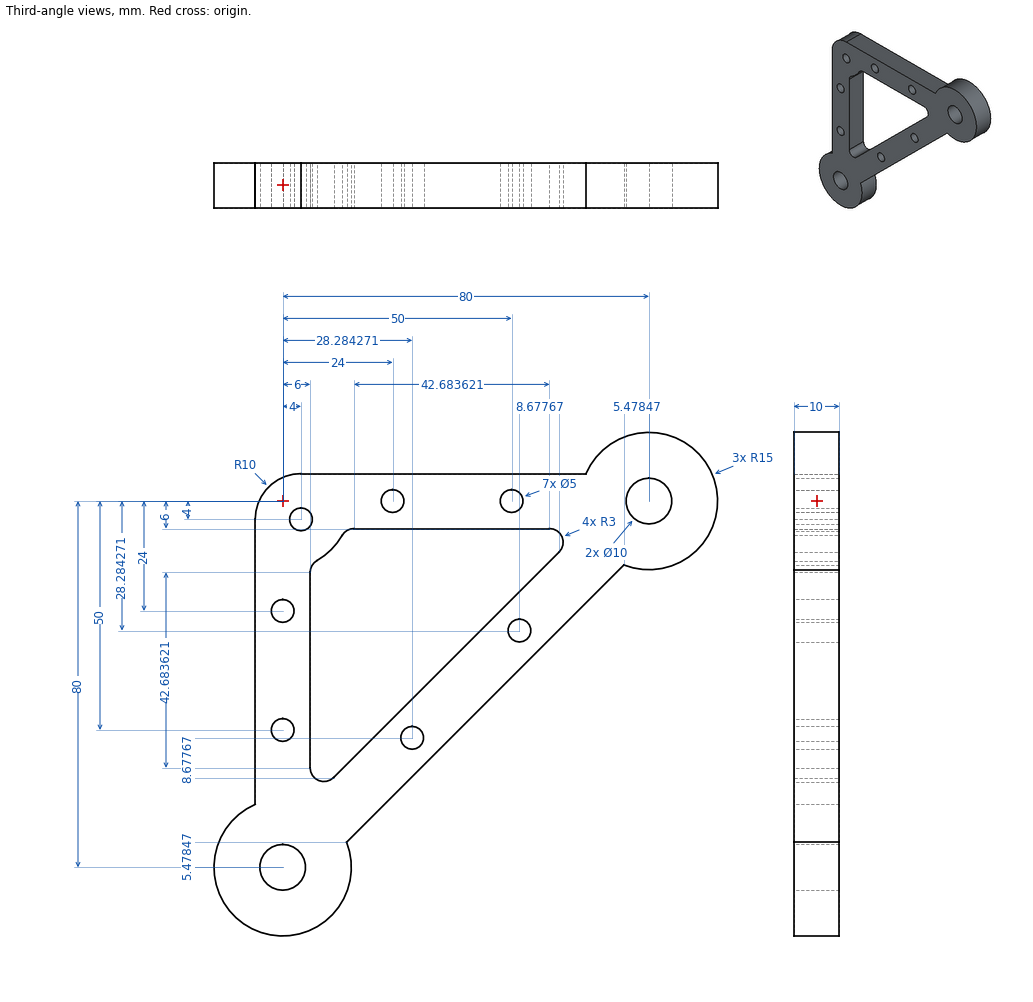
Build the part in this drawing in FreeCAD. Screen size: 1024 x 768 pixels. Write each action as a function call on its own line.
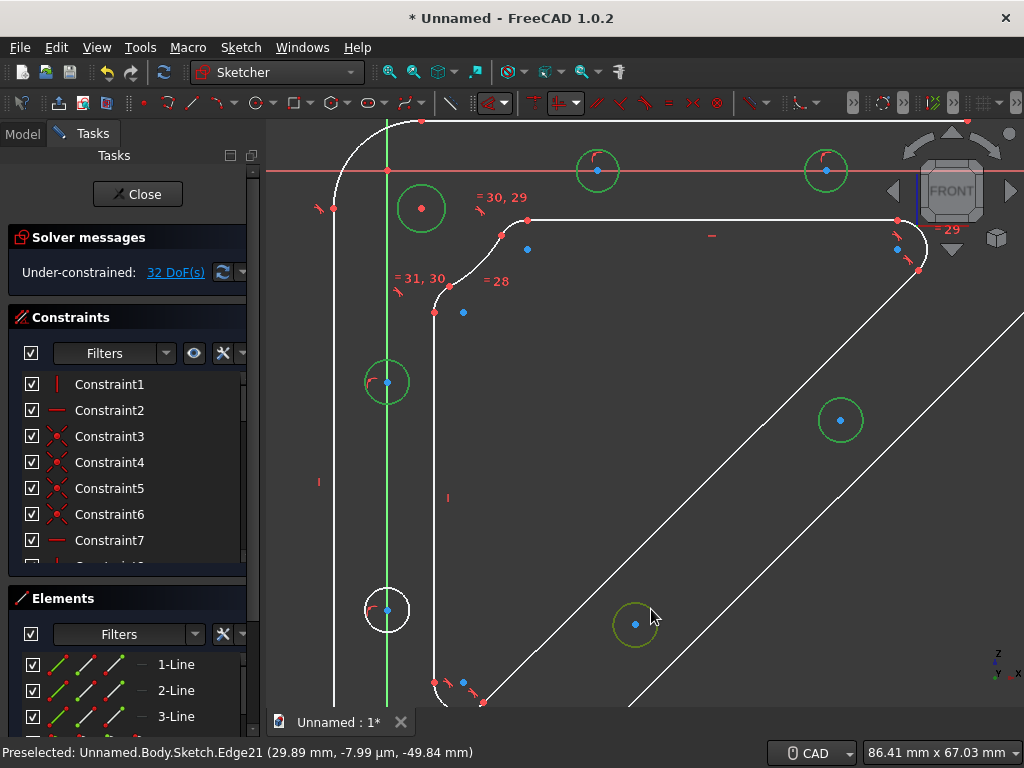
click(403, 594)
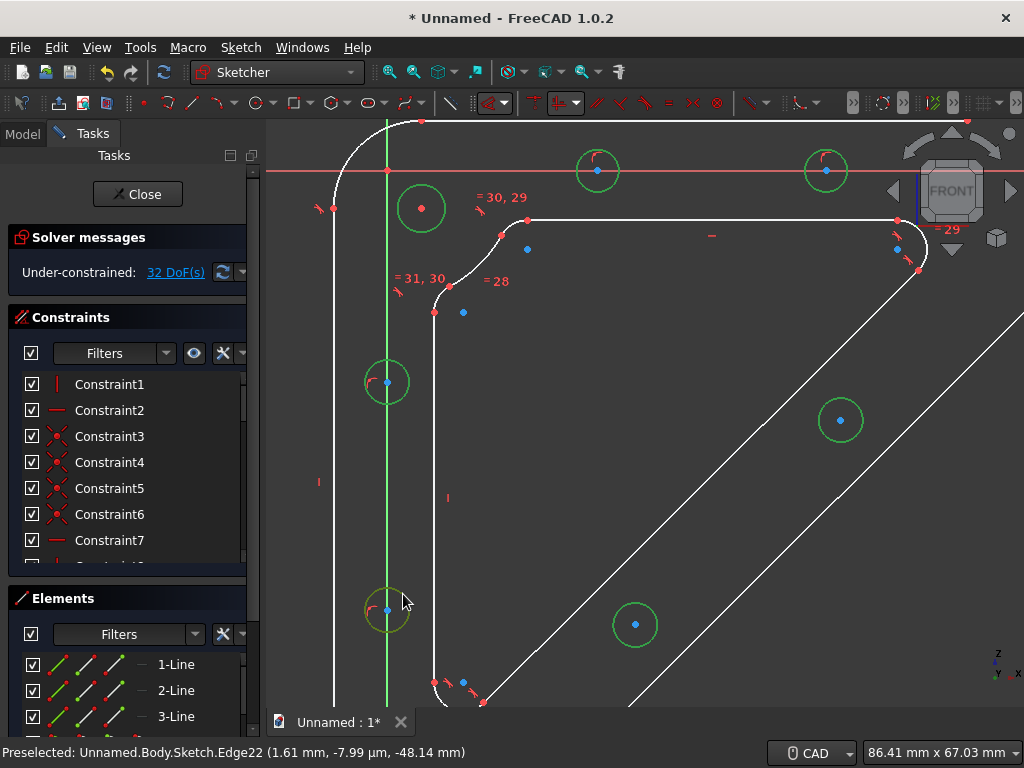
click(670, 104)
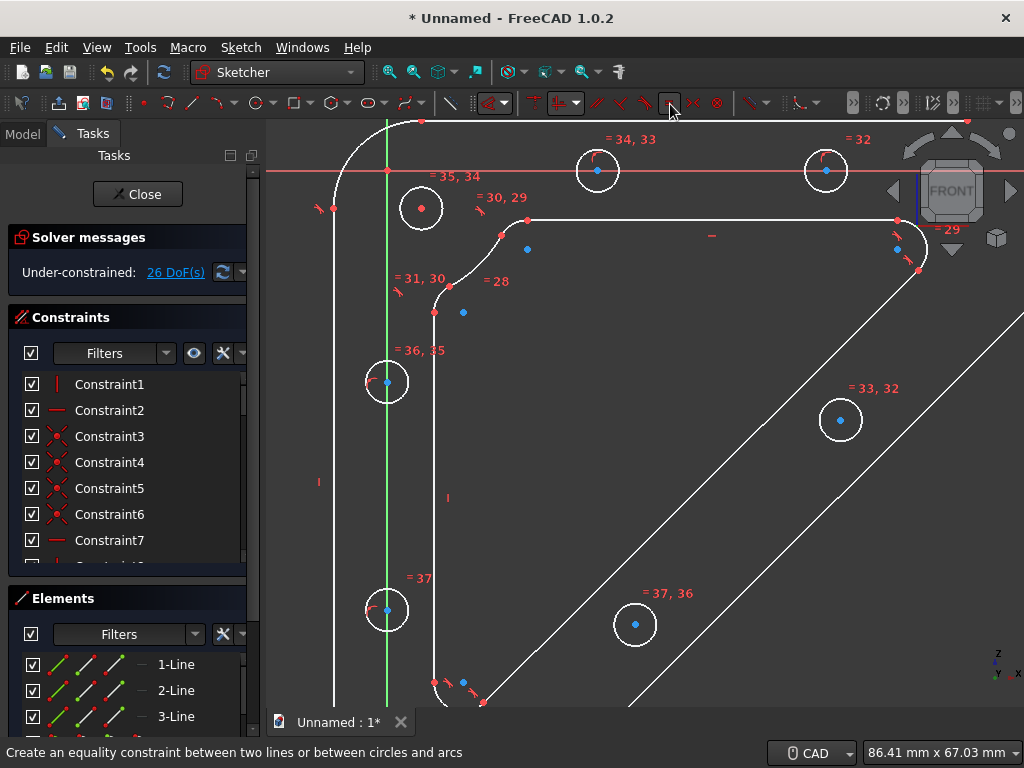
scroll(417, 296, down, 4)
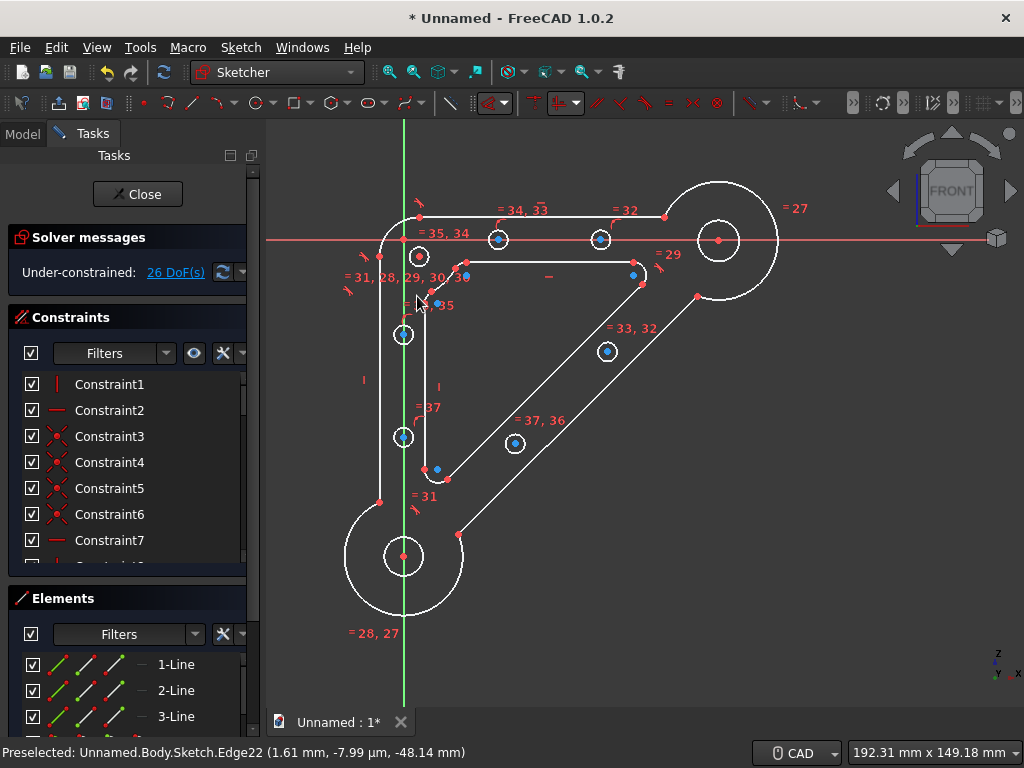
click(733, 226)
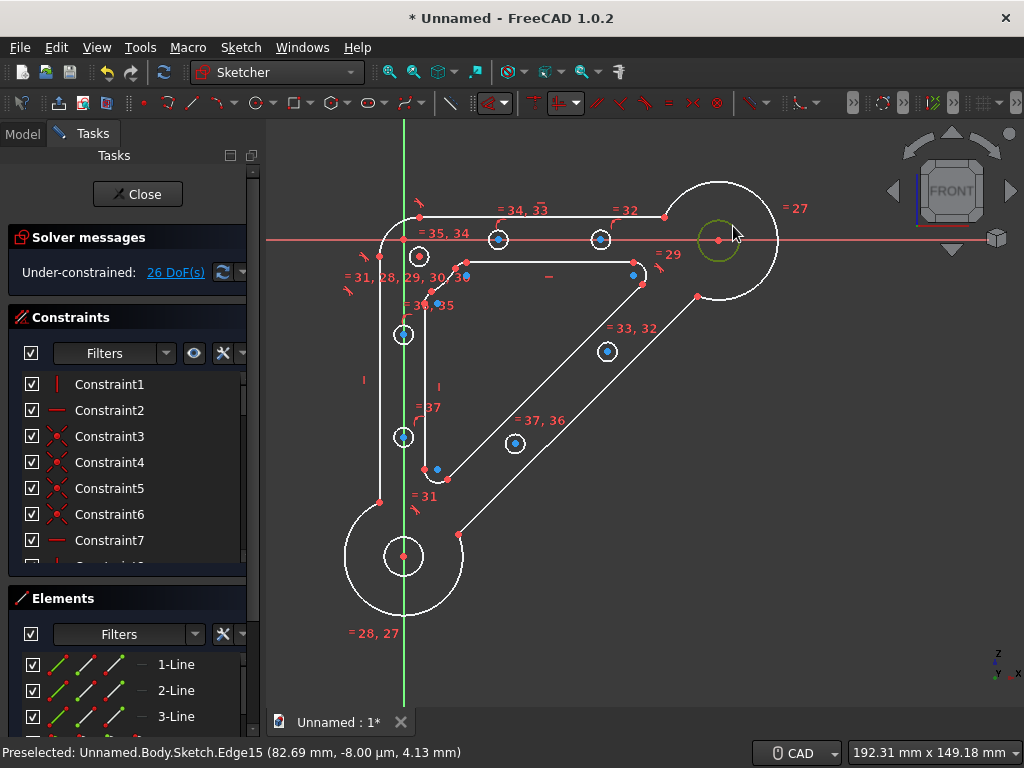
click(417, 543)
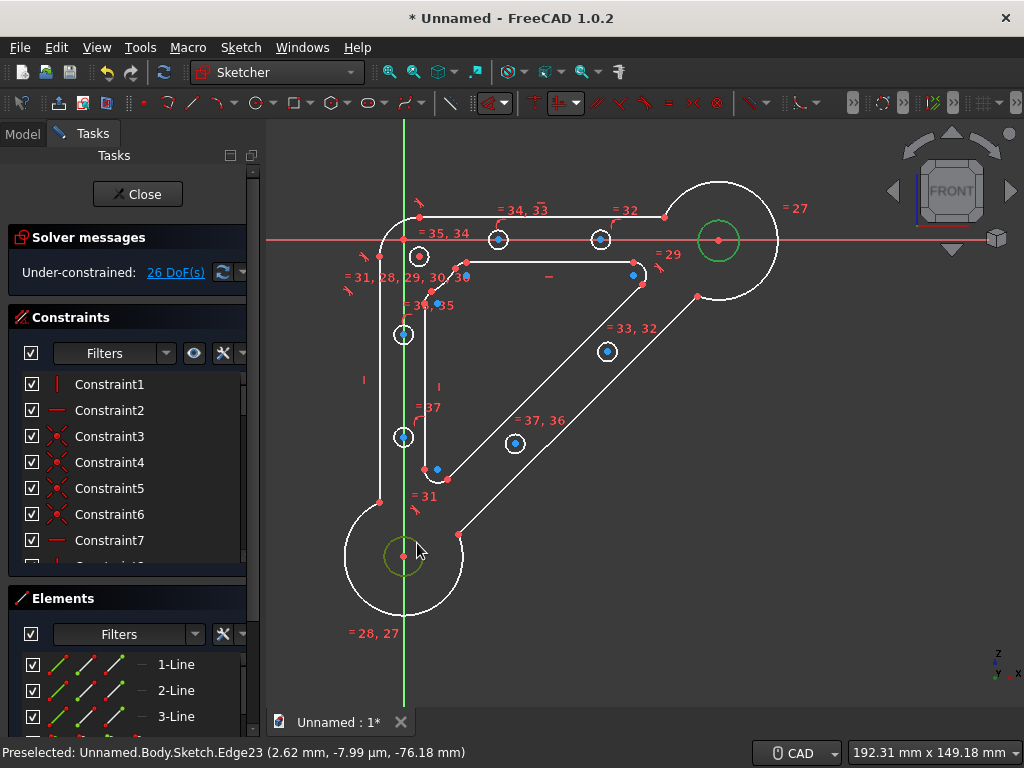
click(670, 104)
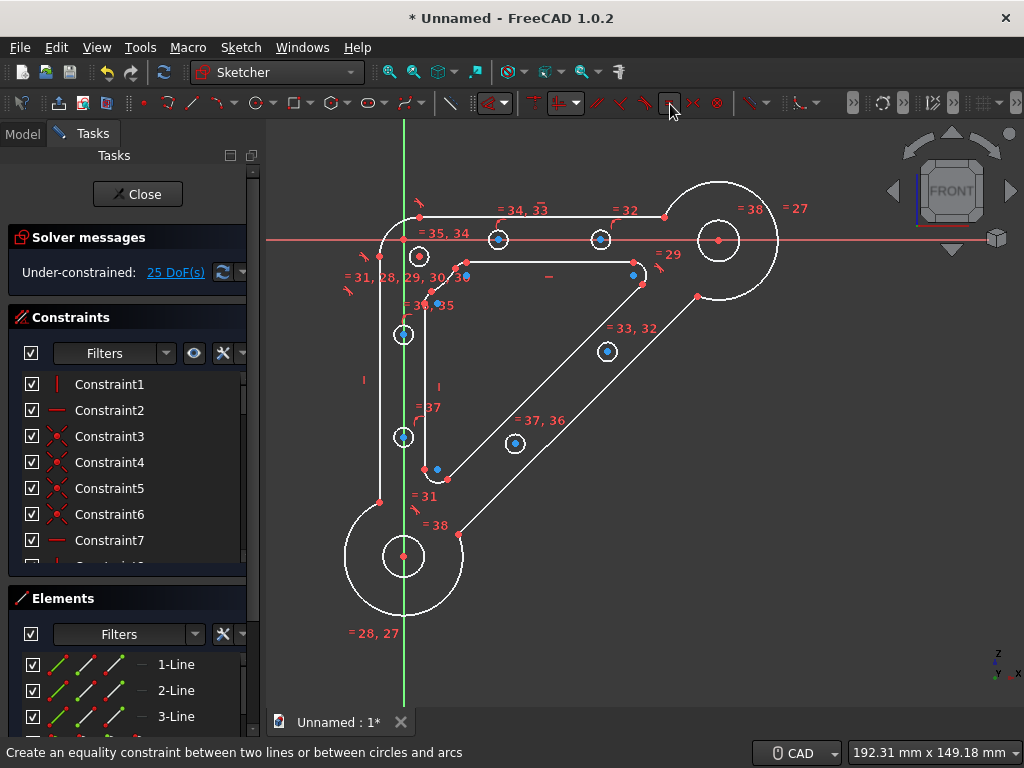
click(719, 241)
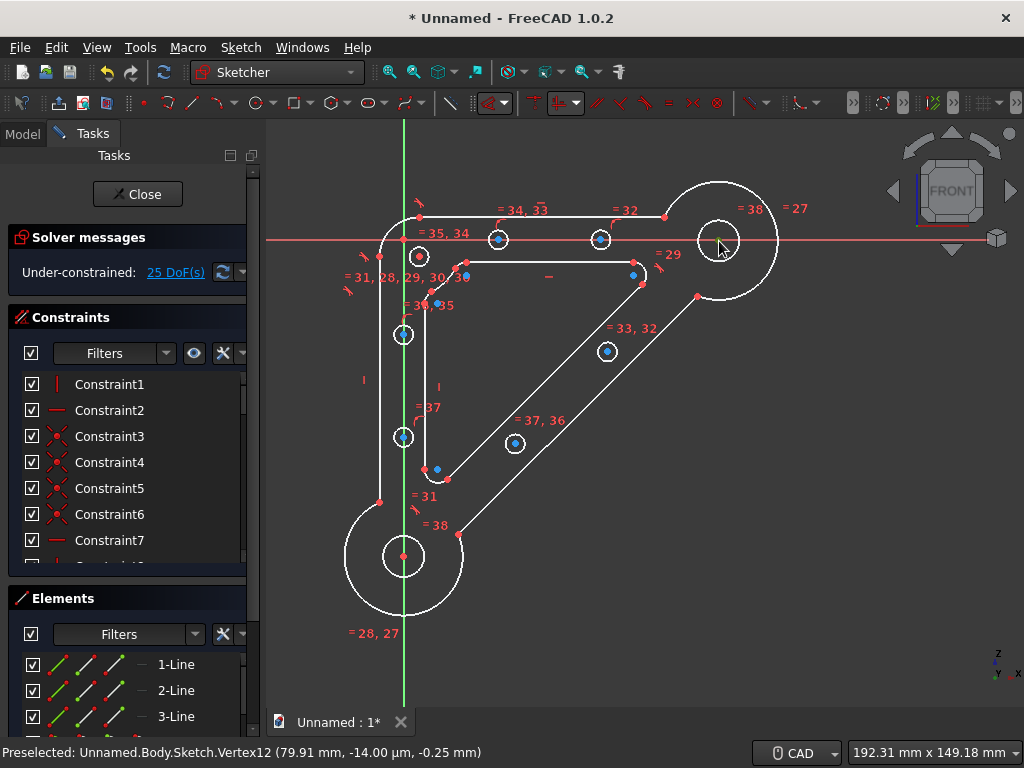
click(334, 240)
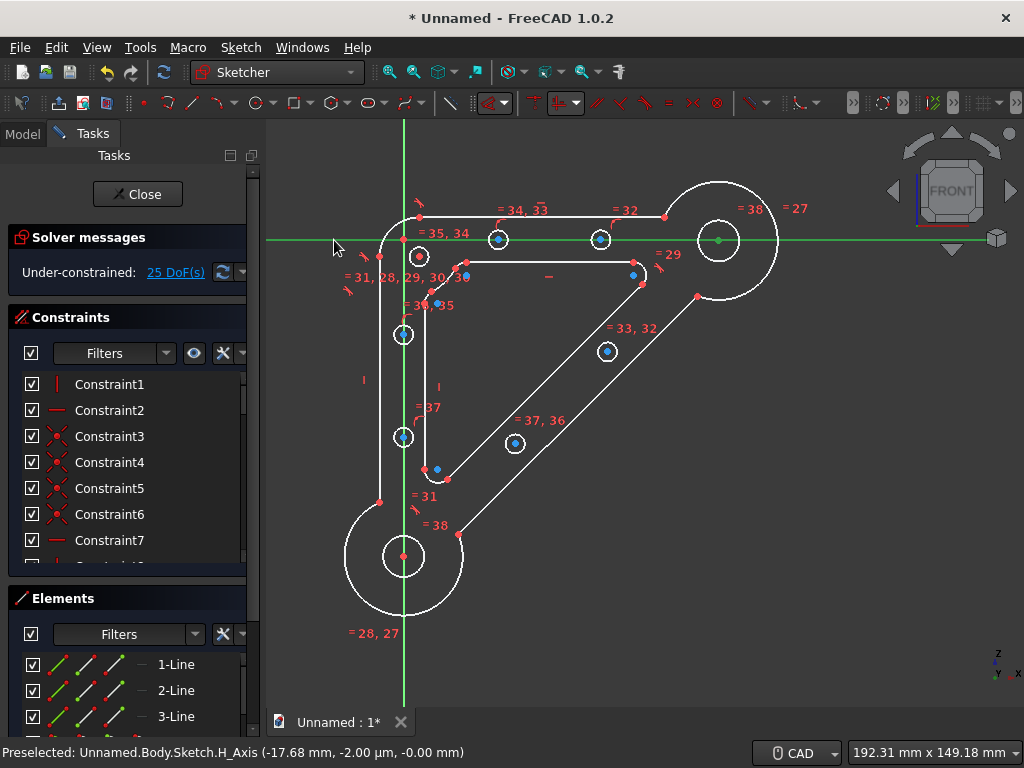
key(c)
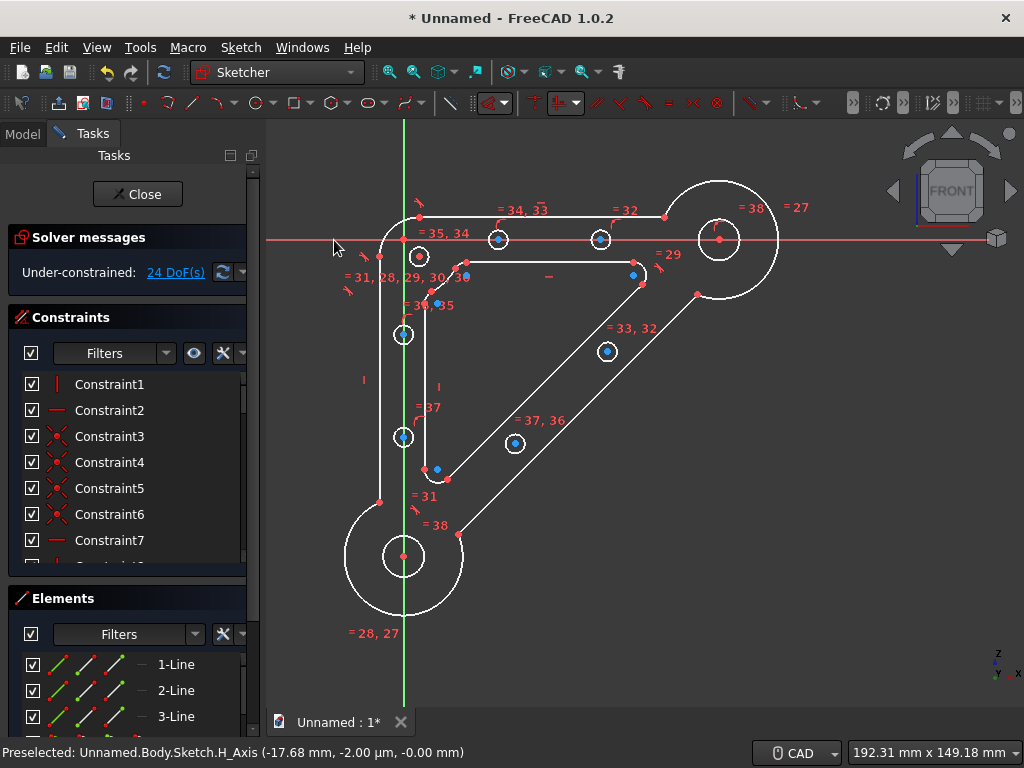
click(404, 557)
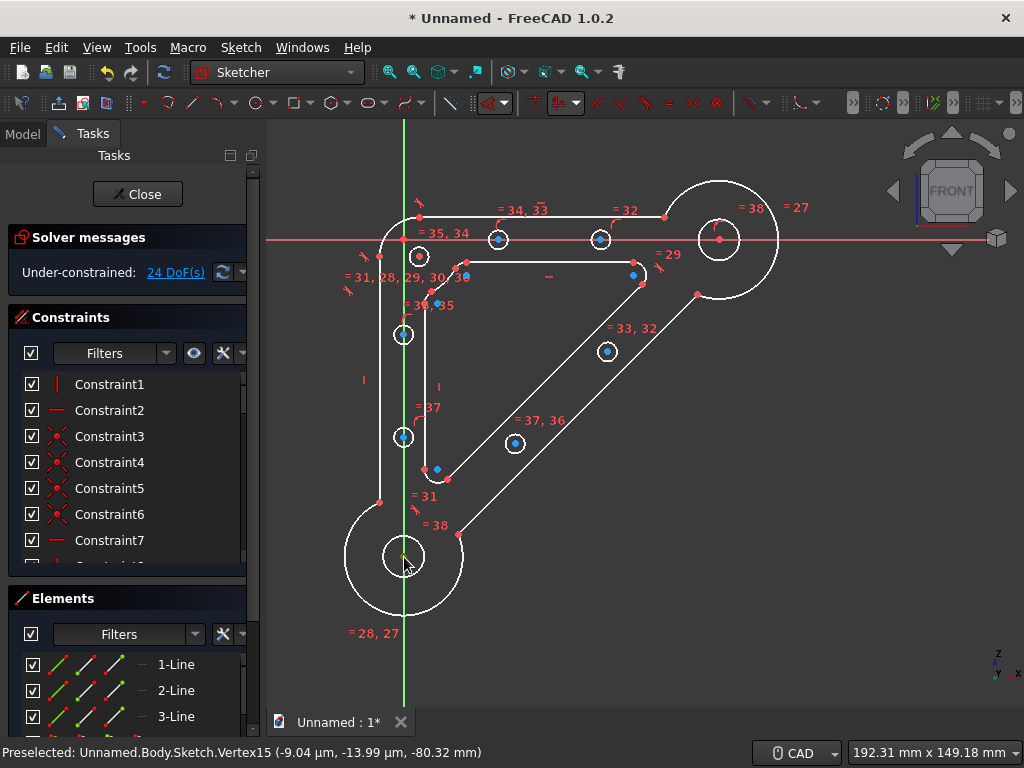
click(404, 185)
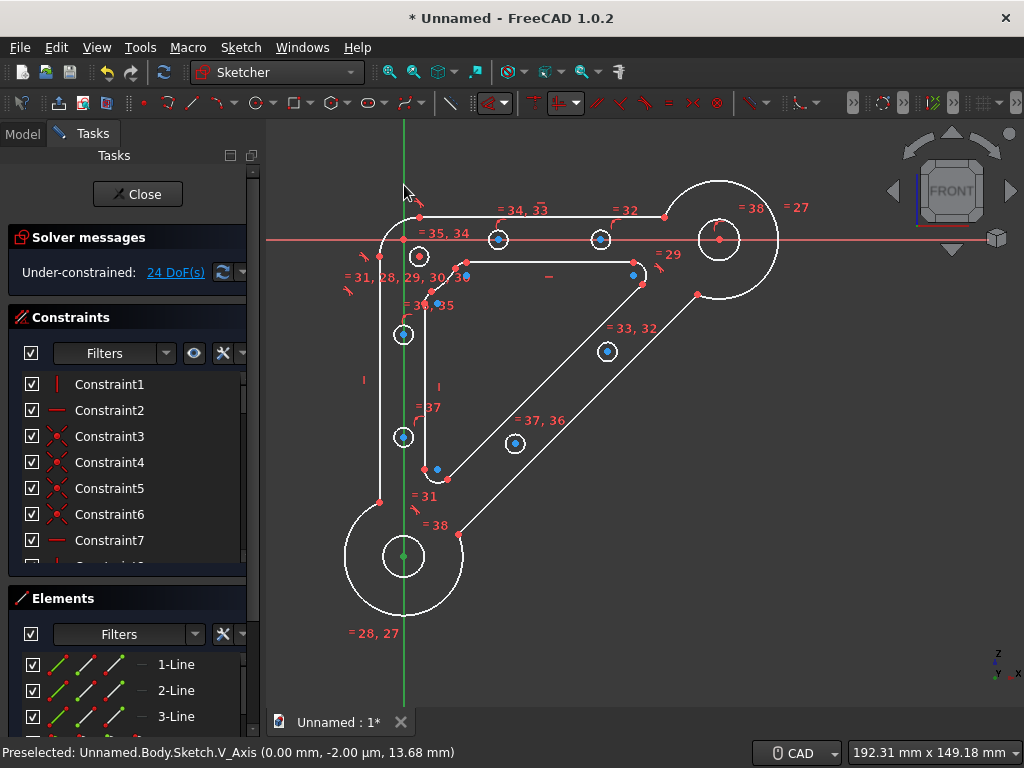
click(534, 104)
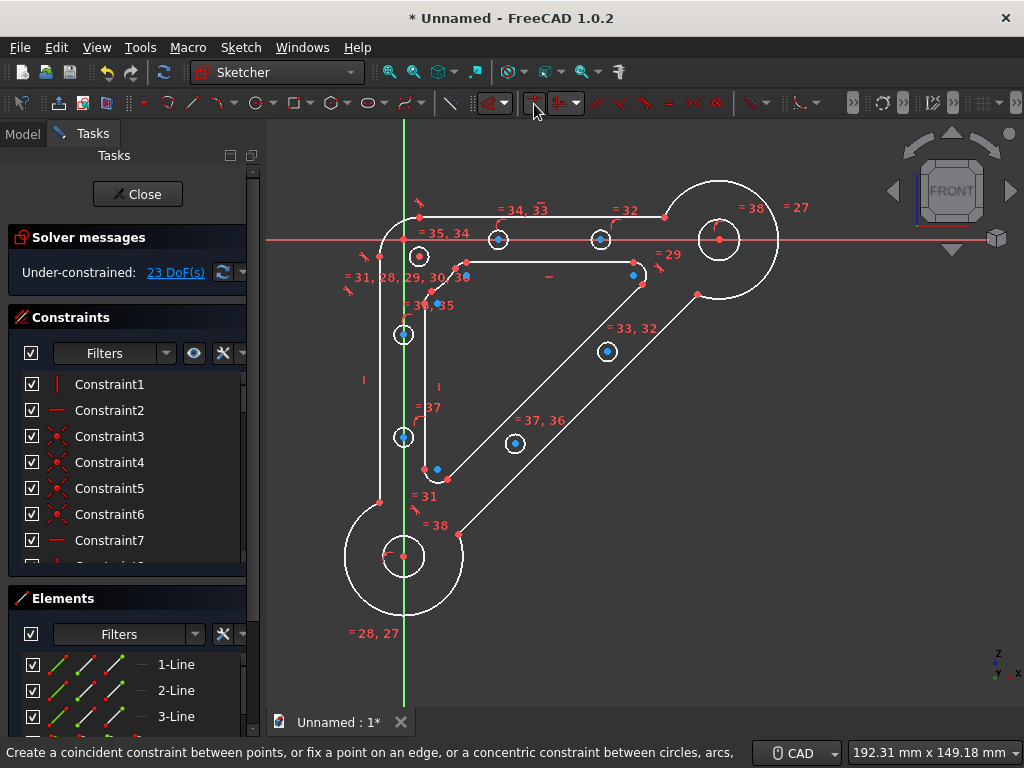
click(488, 104)